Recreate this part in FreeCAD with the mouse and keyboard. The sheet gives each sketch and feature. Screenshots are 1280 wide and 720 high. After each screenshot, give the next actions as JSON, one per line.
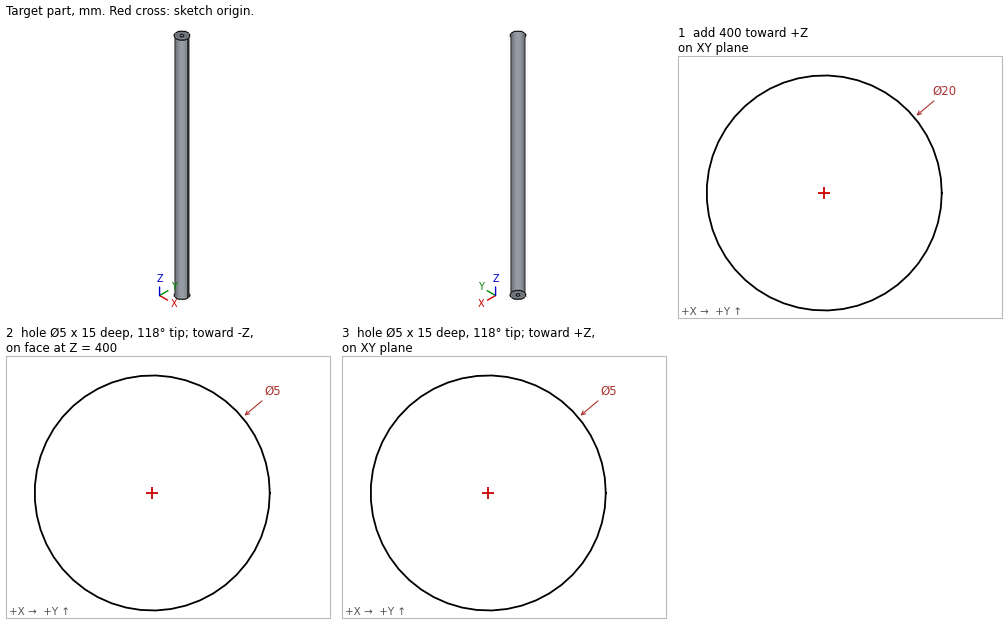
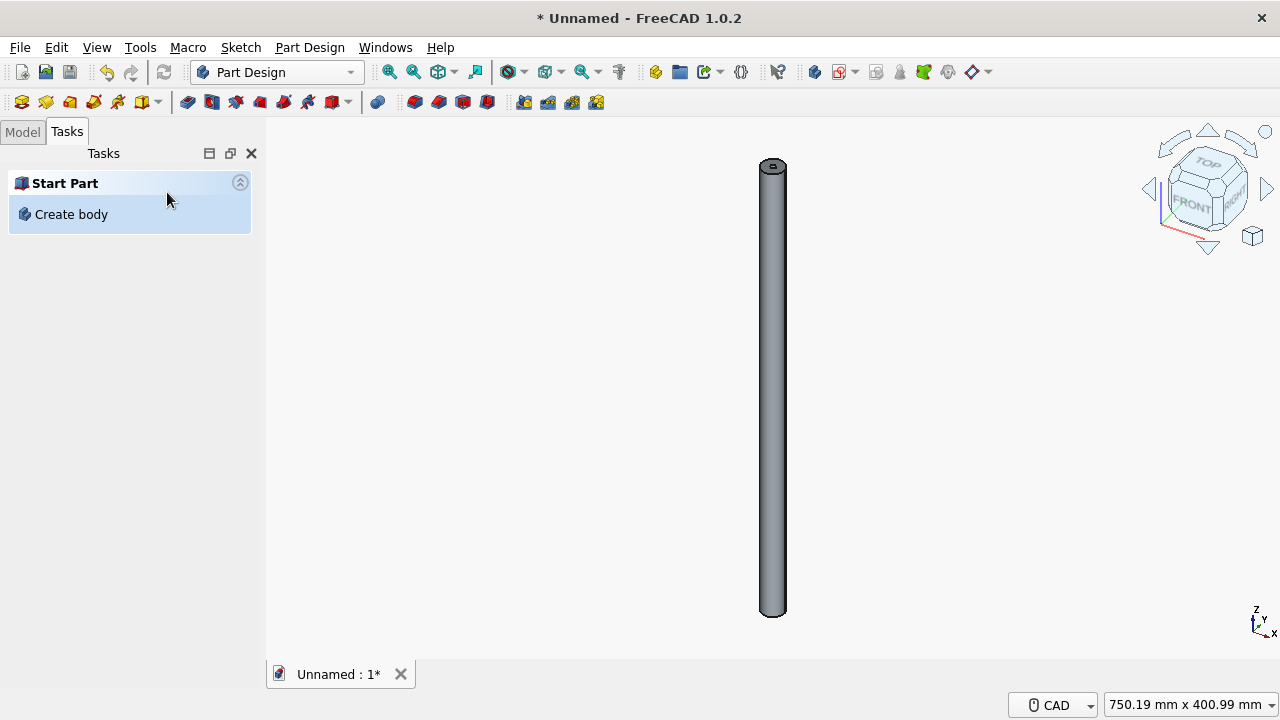
{"action": "key", "text": "0"}